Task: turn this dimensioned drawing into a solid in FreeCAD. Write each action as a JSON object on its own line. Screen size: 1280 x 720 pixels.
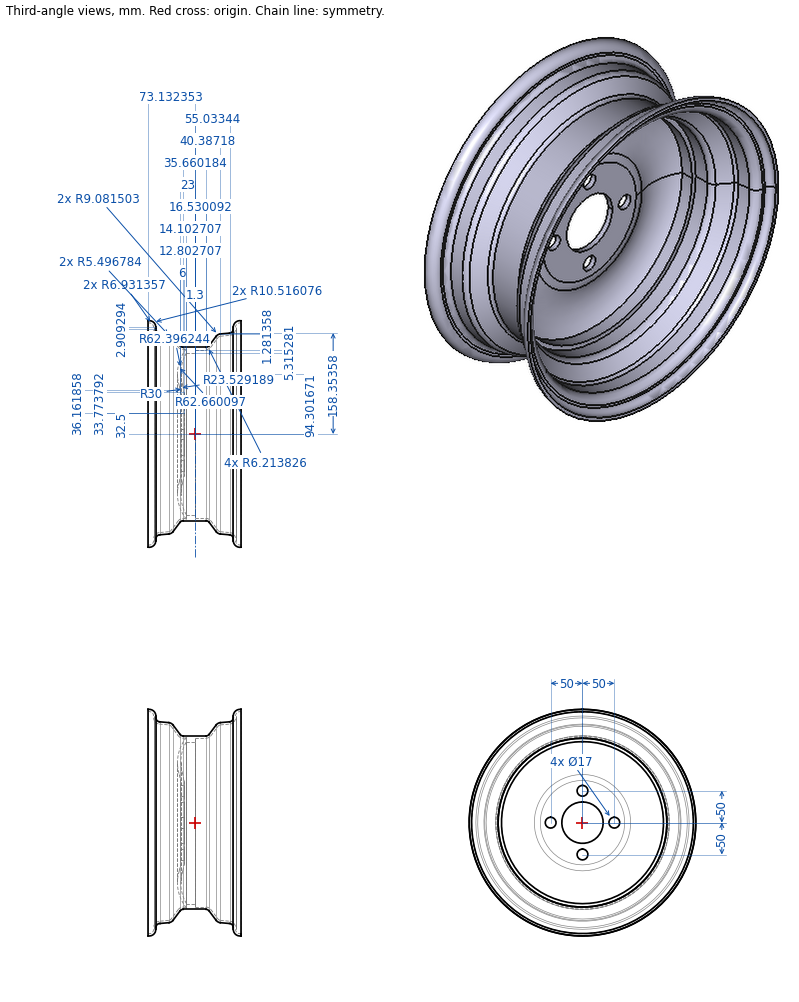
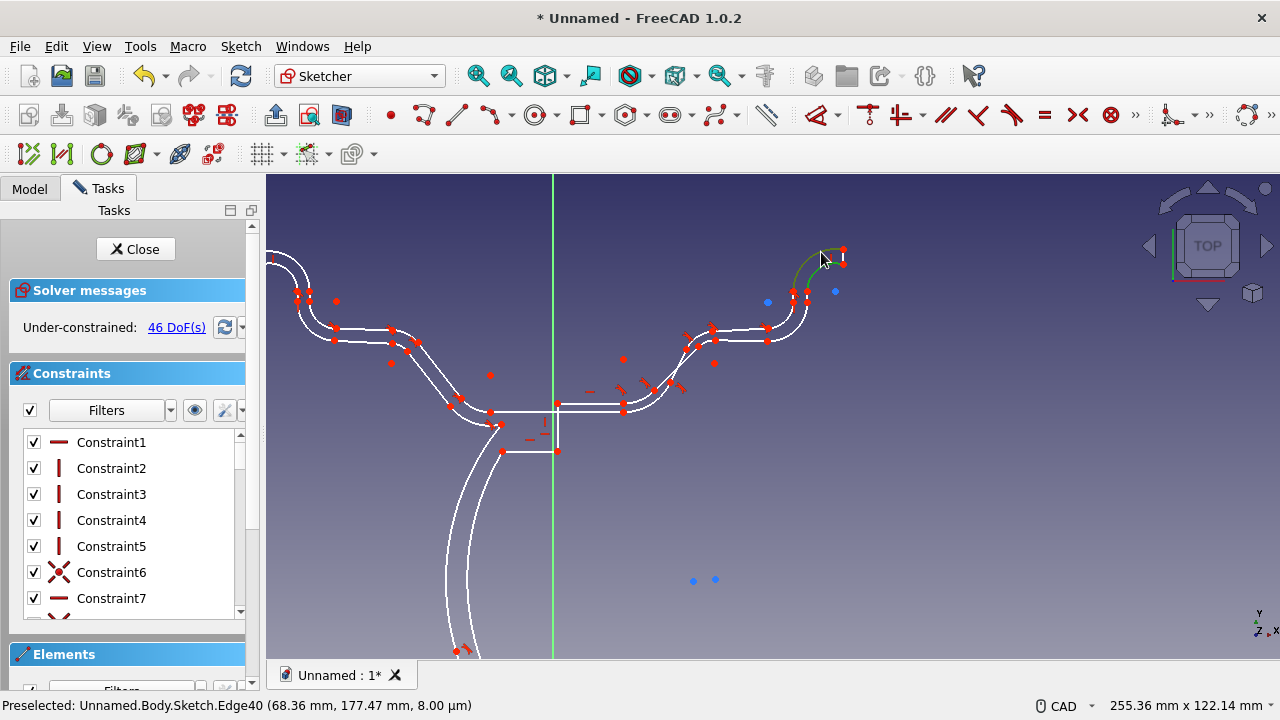
{"action": "key", "text": "c"}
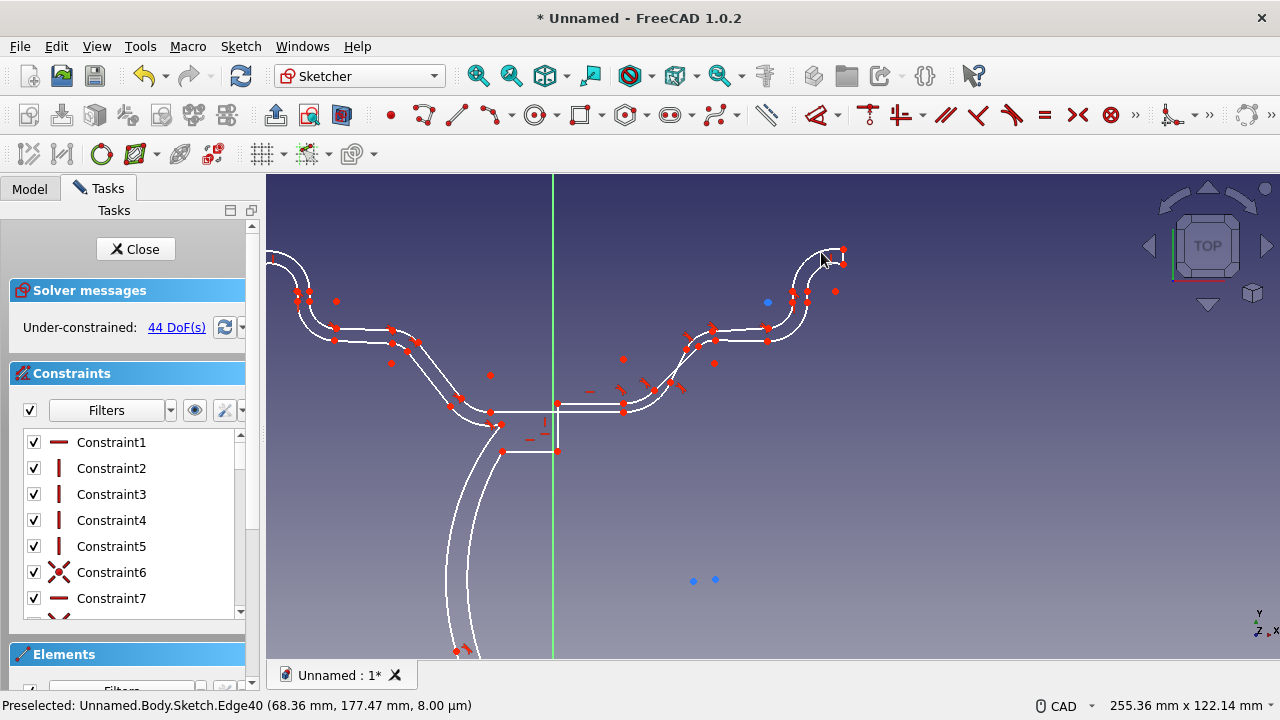
{"action": "left_click", "coordinate": [786, 337]}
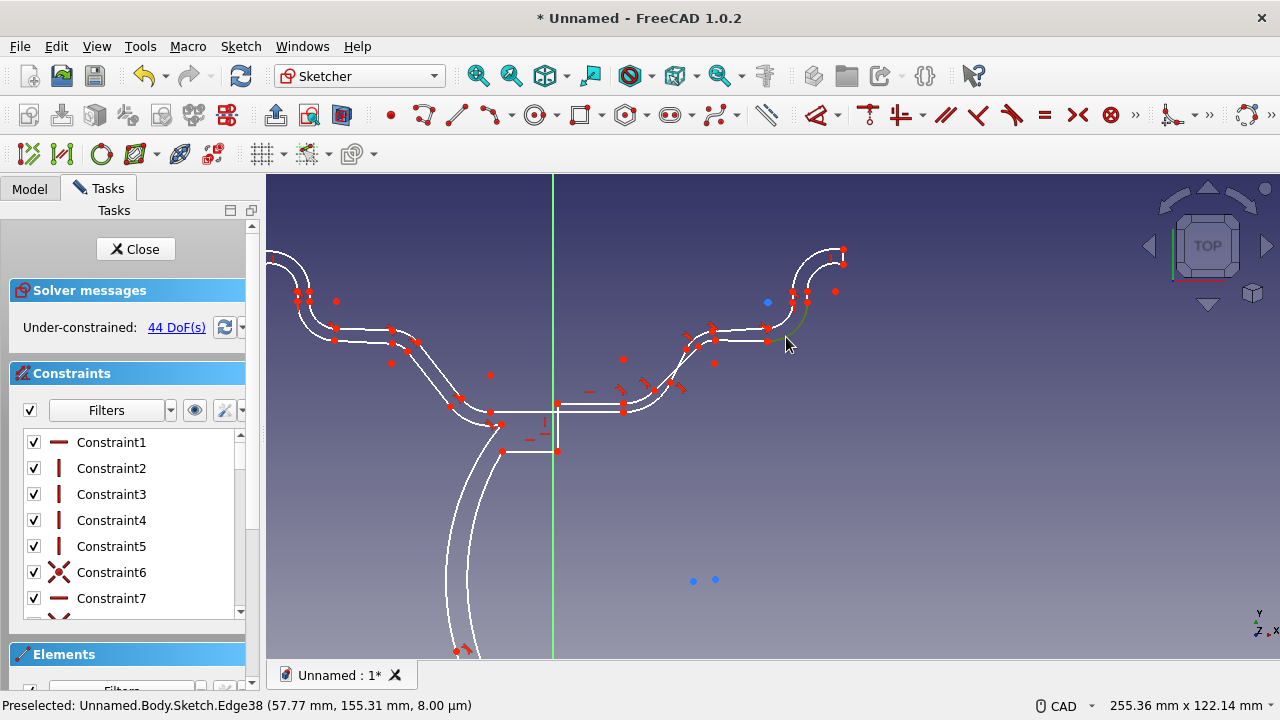
{"action": "left_click", "coordinate": [780, 325]}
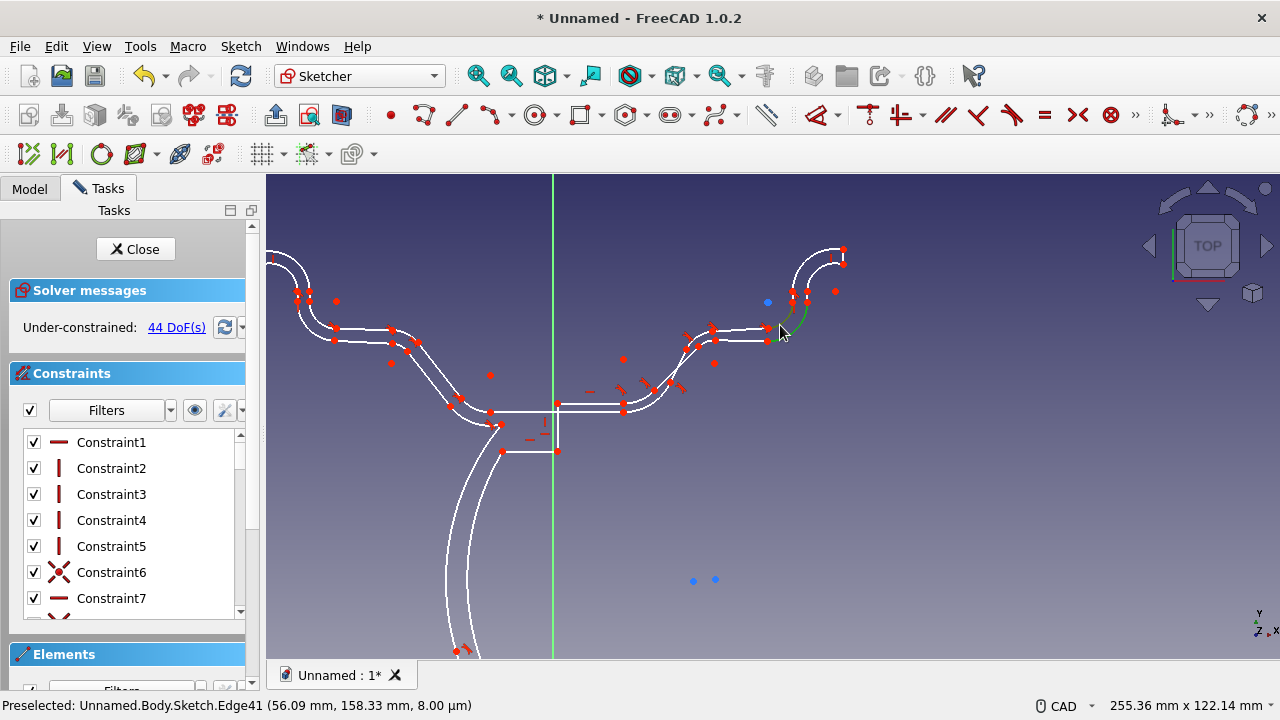
{"action": "left_click", "coordinate": [868, 116]}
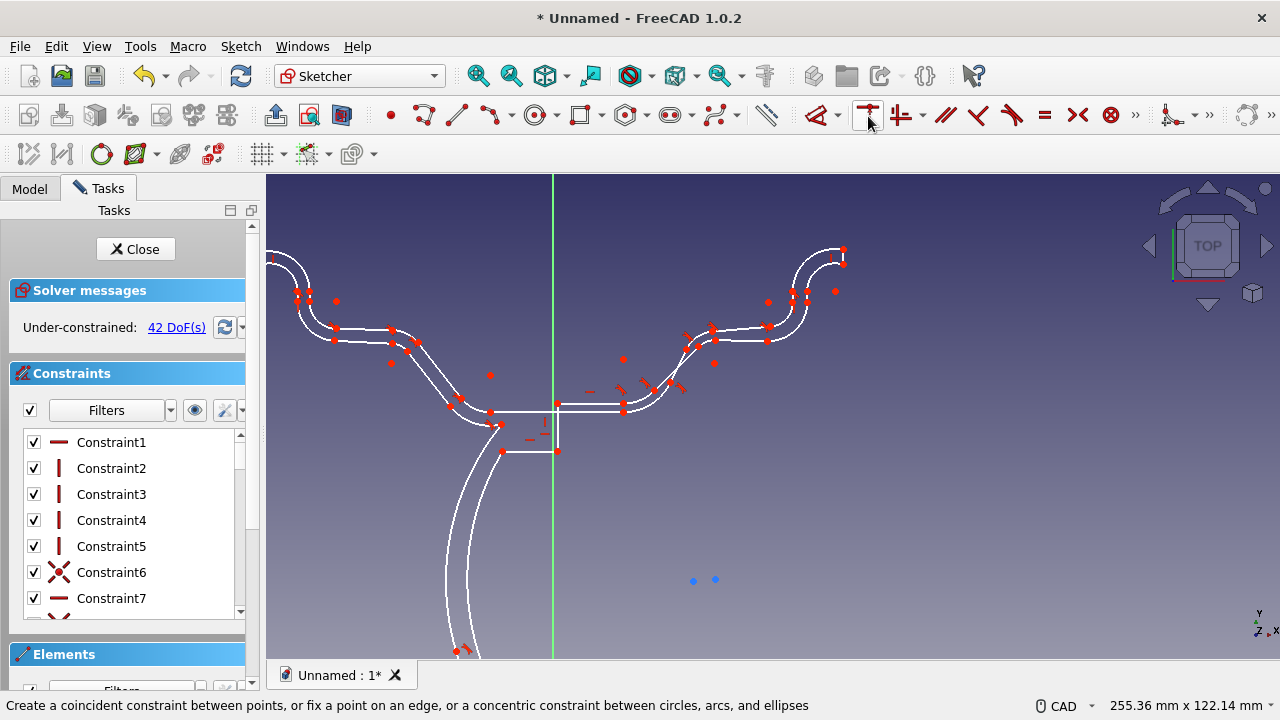
{"action": "scroll", "coordinate": [641, 409], "scroll_direction": "up", "scroll_amount": 3}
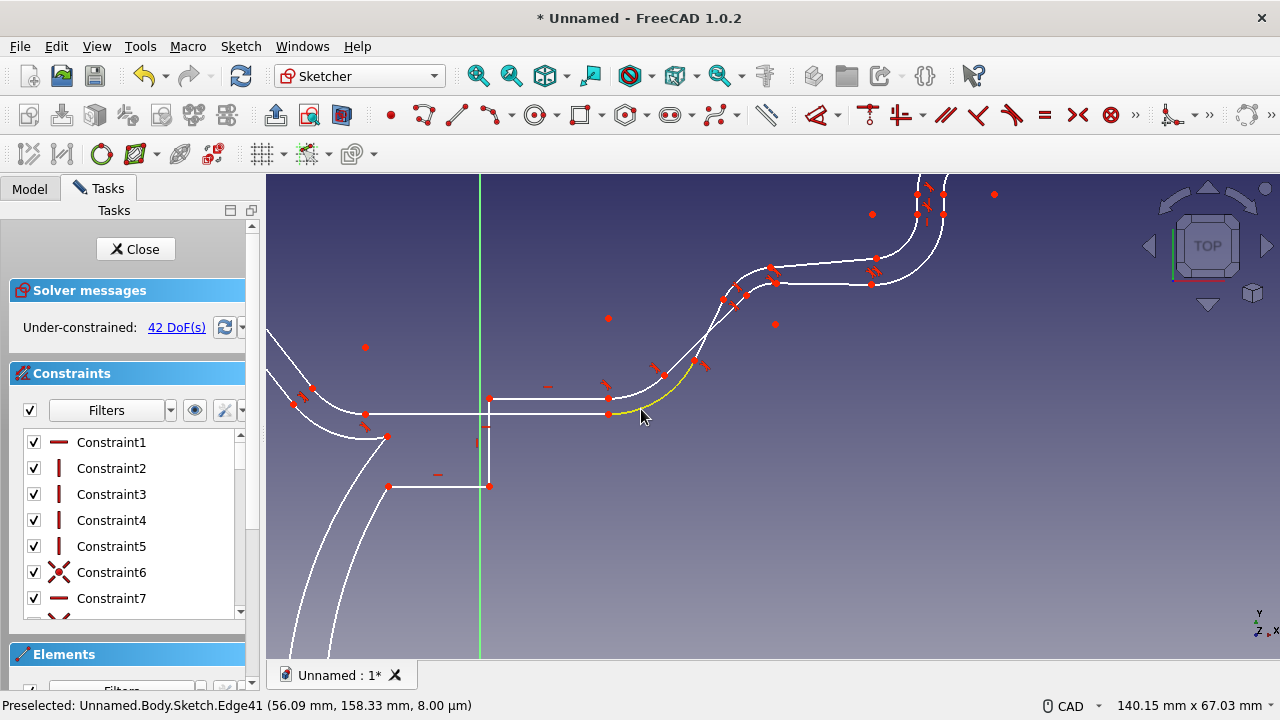
{"action": "left_click", "coordinate": [640, 409]}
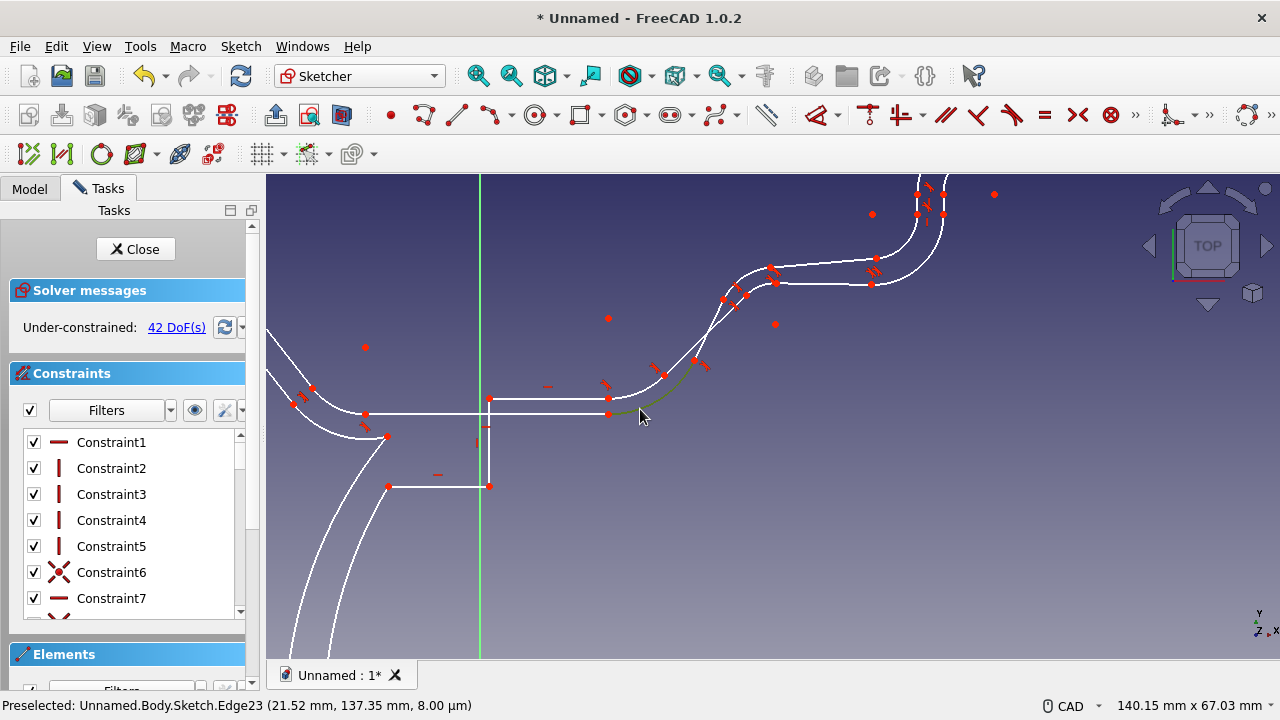
{"action": "left_click", "coordinate": [326, 401]}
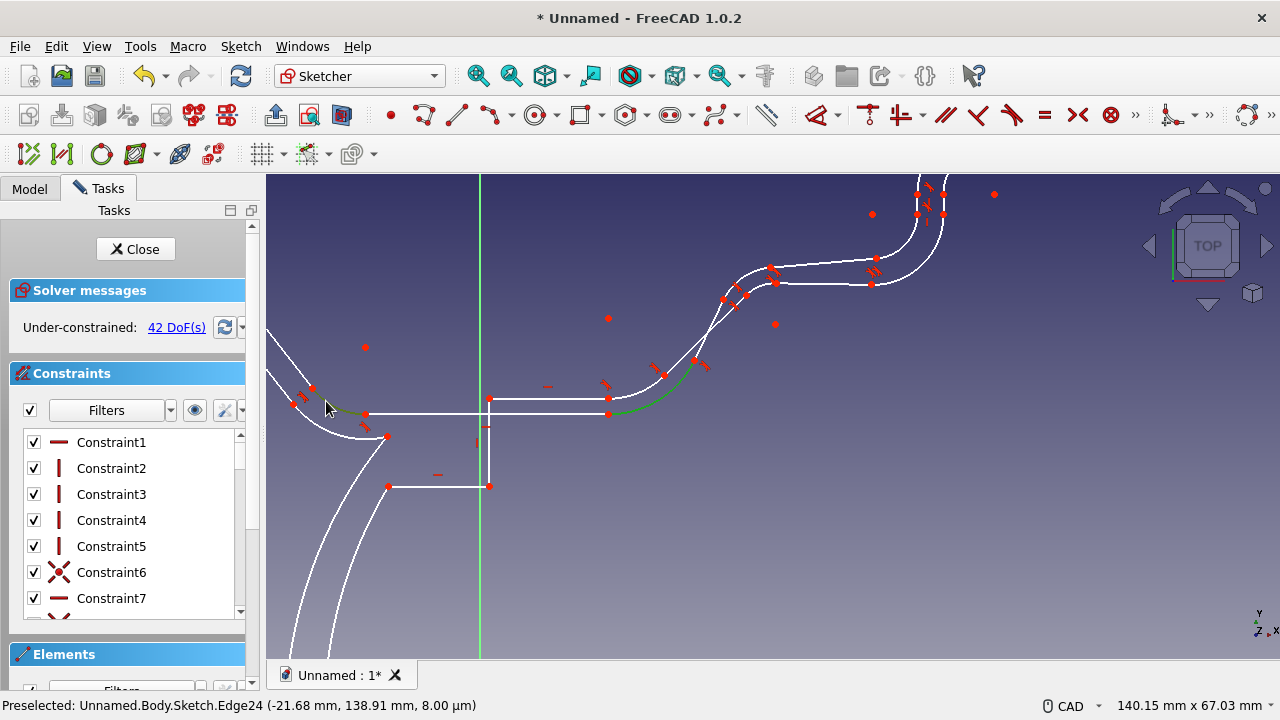
{"action": "scroll", "coordinate": [778, 304], "scroll_direction": "down", "scroll_amount": 7}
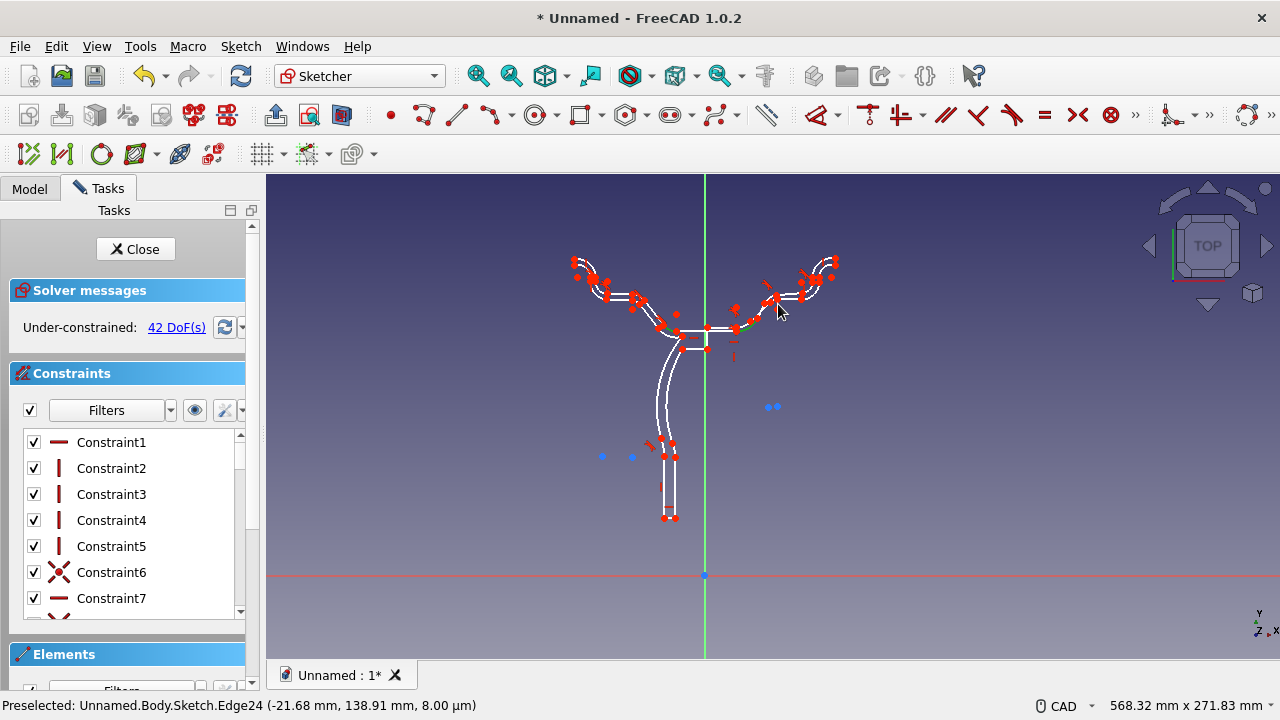
{"action": "scroll", "coordinate": [597, 287], "scroll_direction": "up", "scroll_amount": 5}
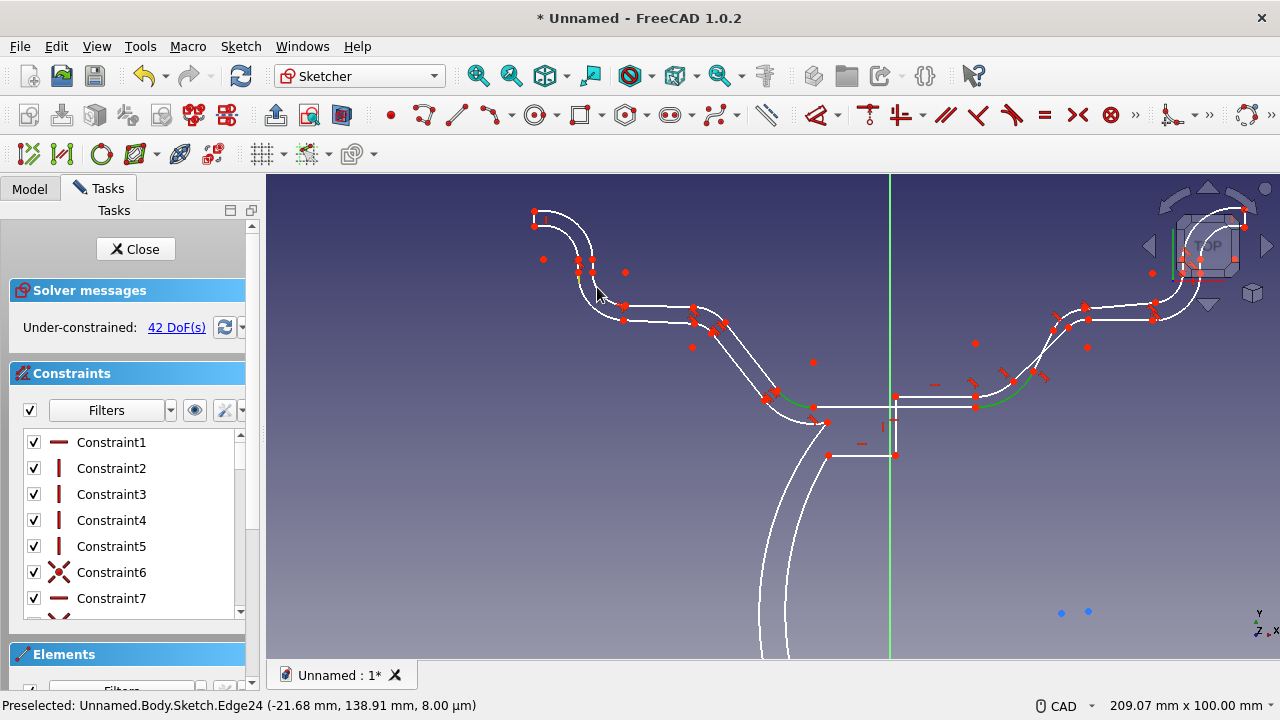
{"action": "left_click", "coordinate": [596, 287]}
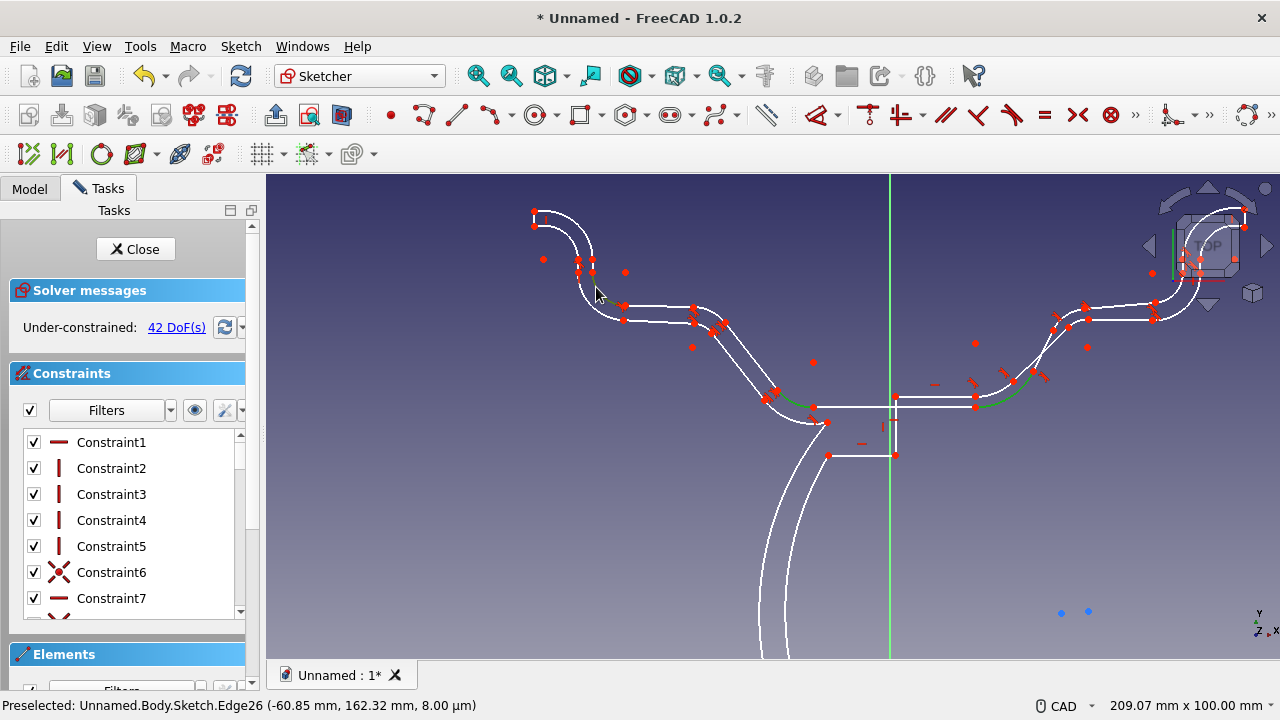
{"action": "scroll", "coordinate": [597, 287], "scroll_direction": "down", "scroll_amount": 5}